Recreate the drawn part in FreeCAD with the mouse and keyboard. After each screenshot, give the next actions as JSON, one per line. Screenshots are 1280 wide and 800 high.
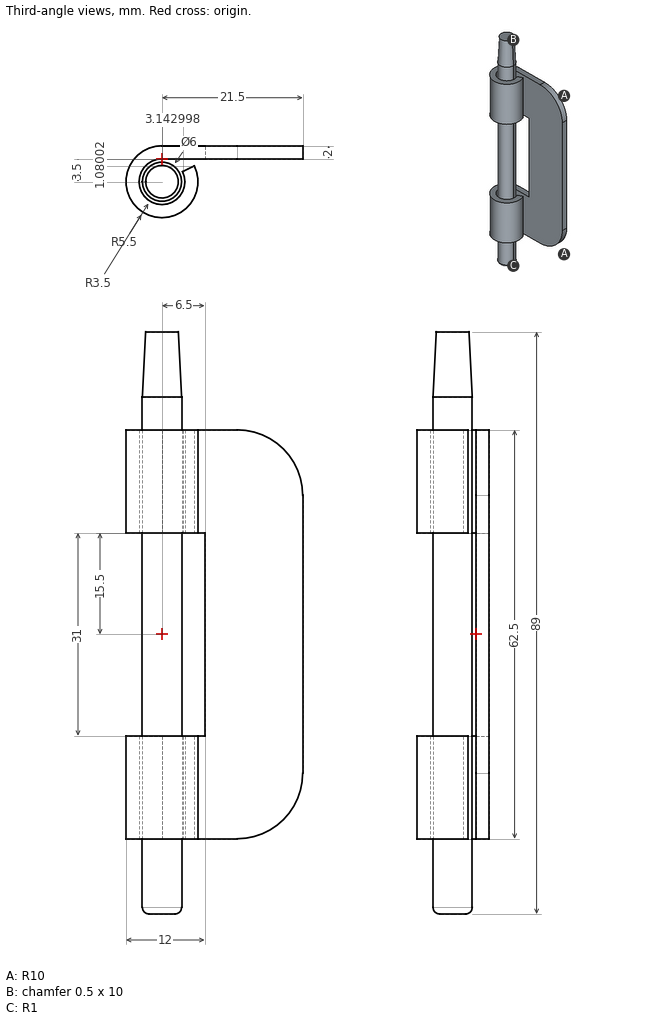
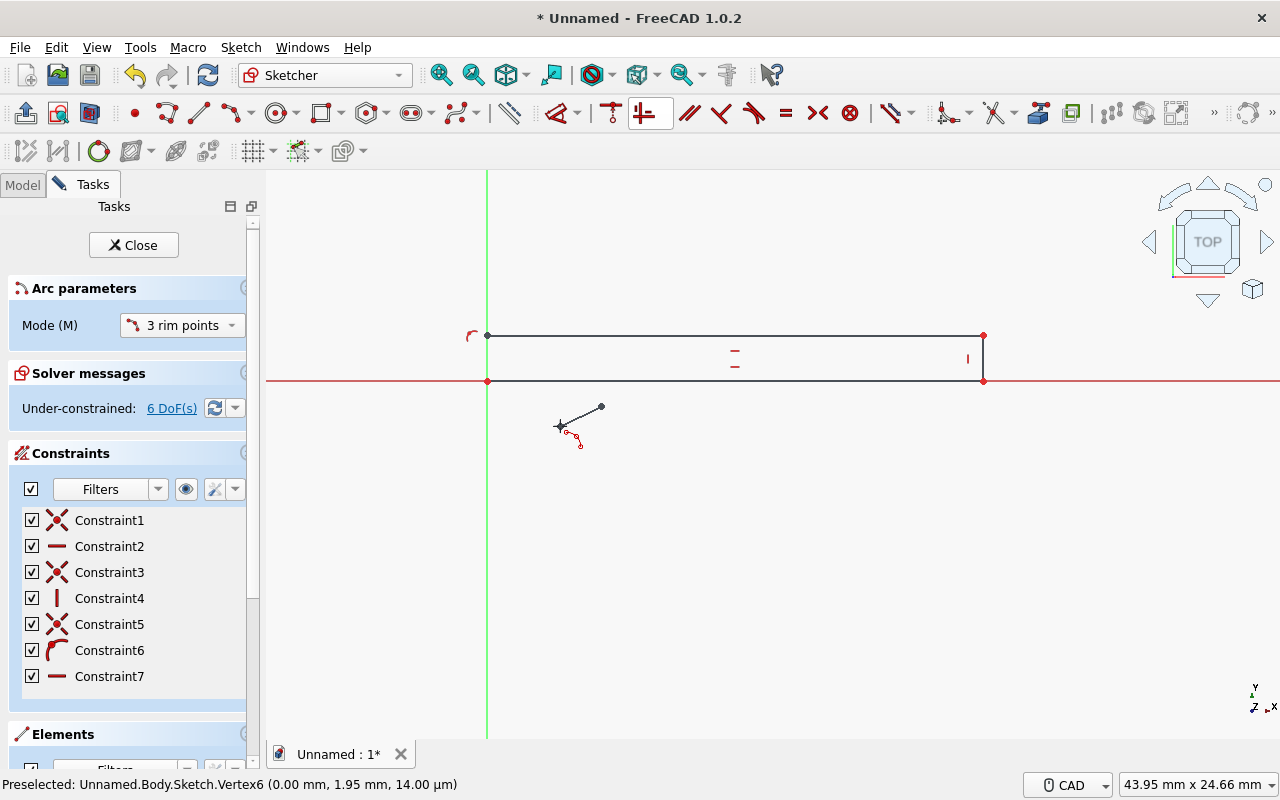
{"action": "left_click", "coordinate": [487, 336]}
{"action": "left_click", "coordinate": [601, 407]}
{"action": "left_click", "coordinate": [420, 569]}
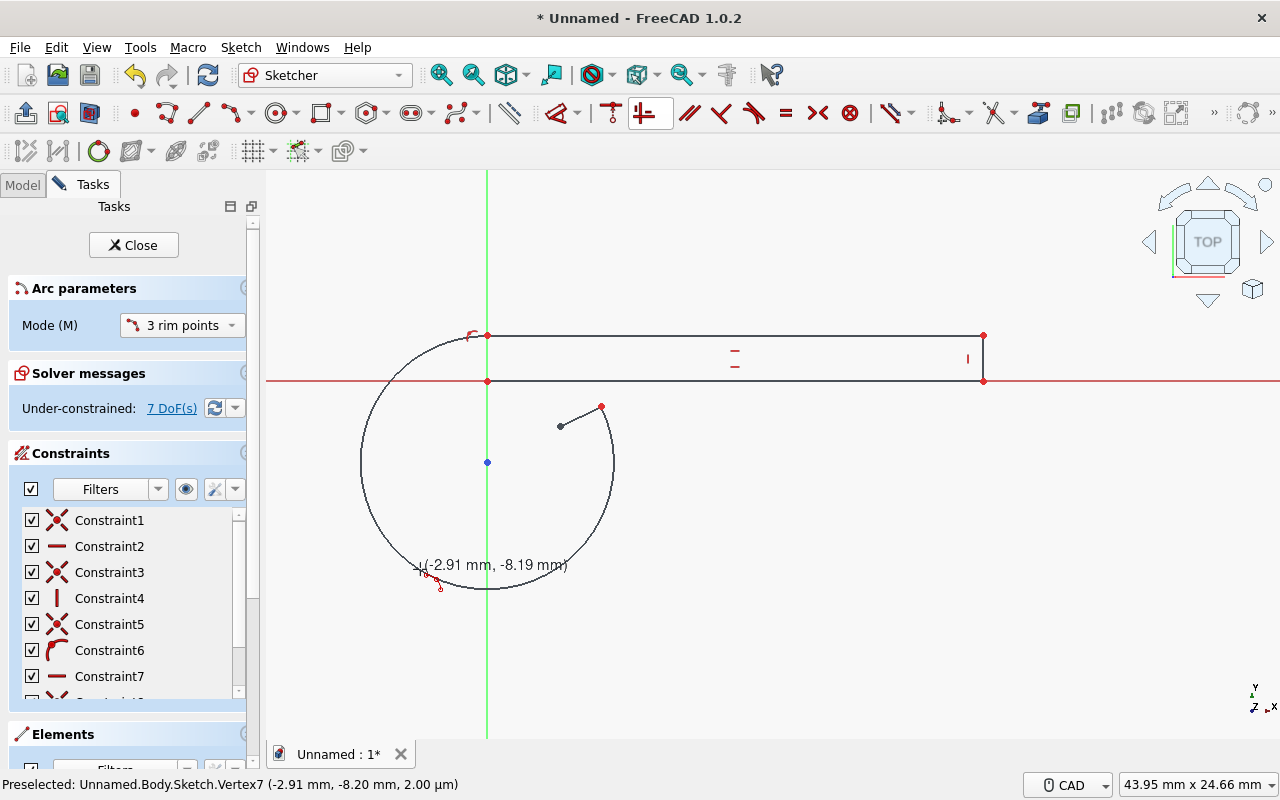
{"action": "left_click", "coordinate": [560, 427]}
{"action": "left_click", "coordinate": [487, 381]}
{"action": "left_click", "coordinate": [444, 530]}
{"action": "key", "text": "Escape"}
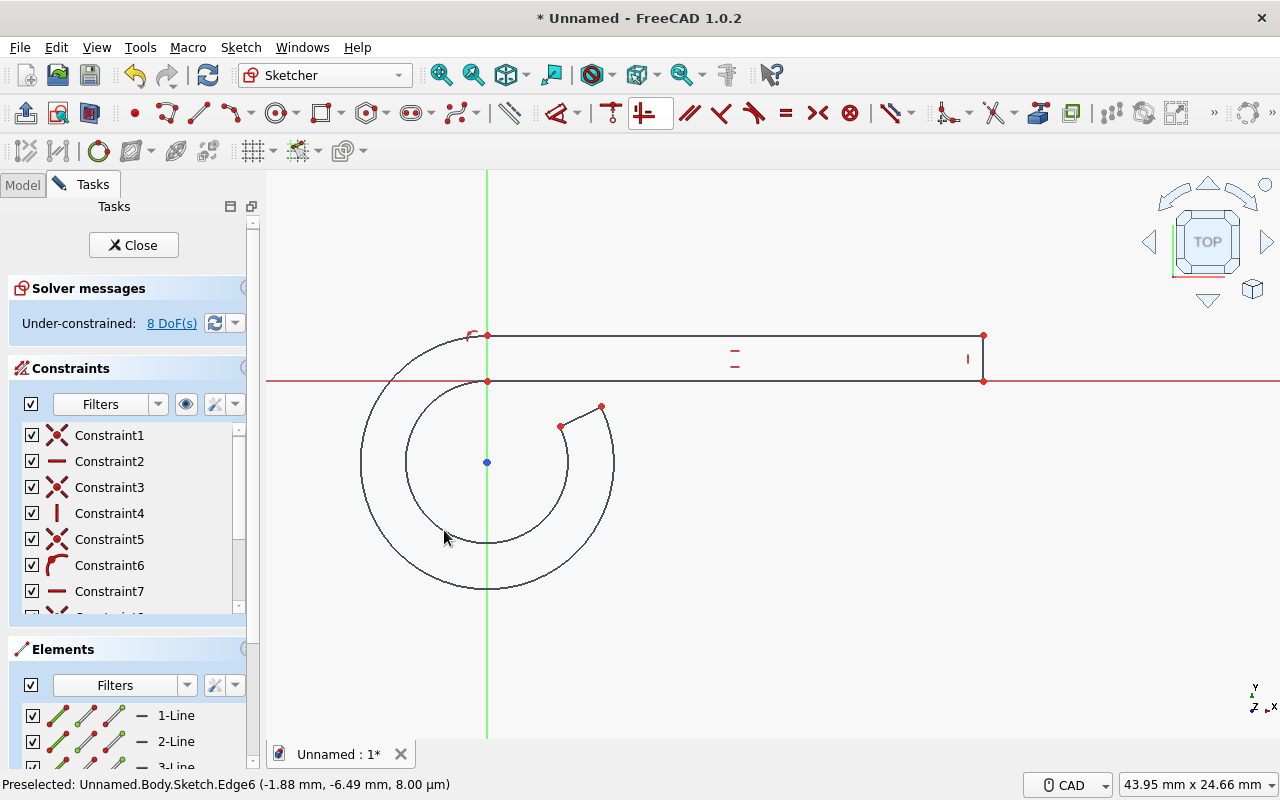
{"action": "left_click", "coordinate": [636, 381]}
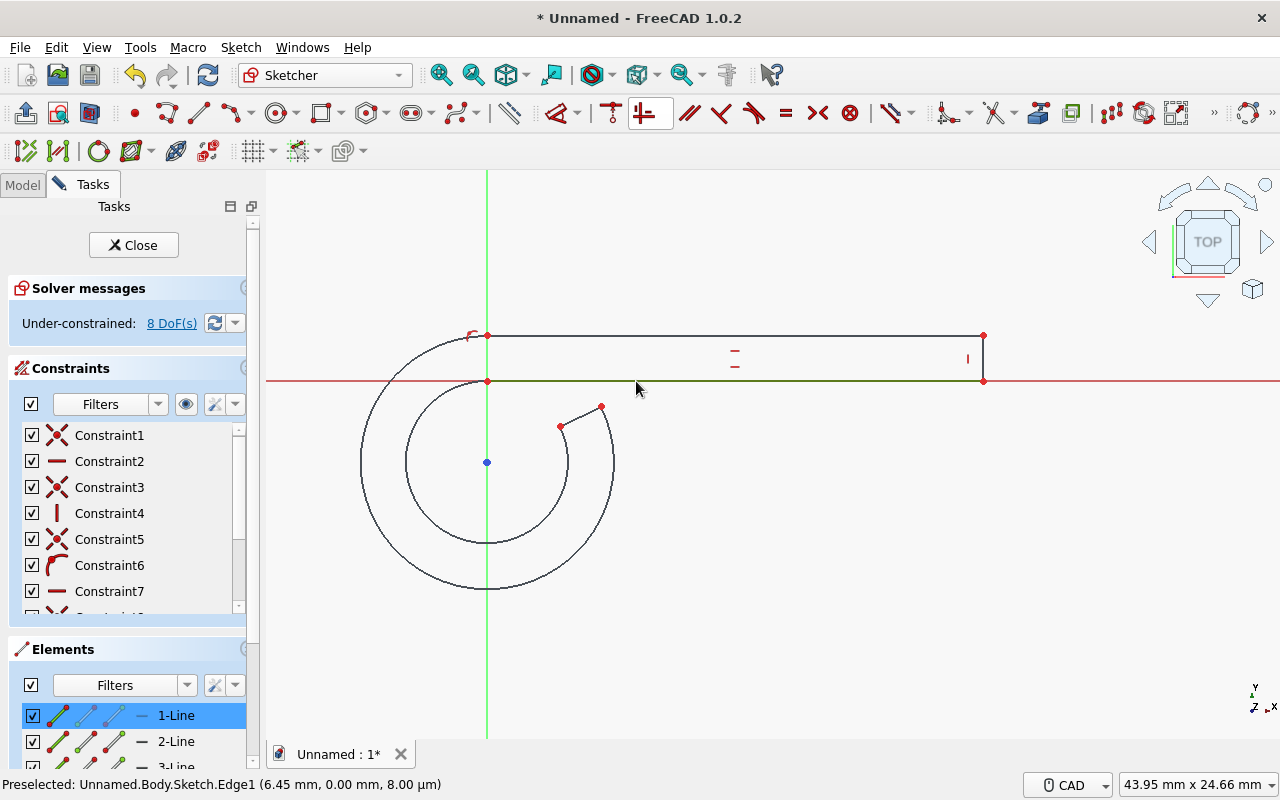
{"action": "left_click", "coordinate": [406, 460]}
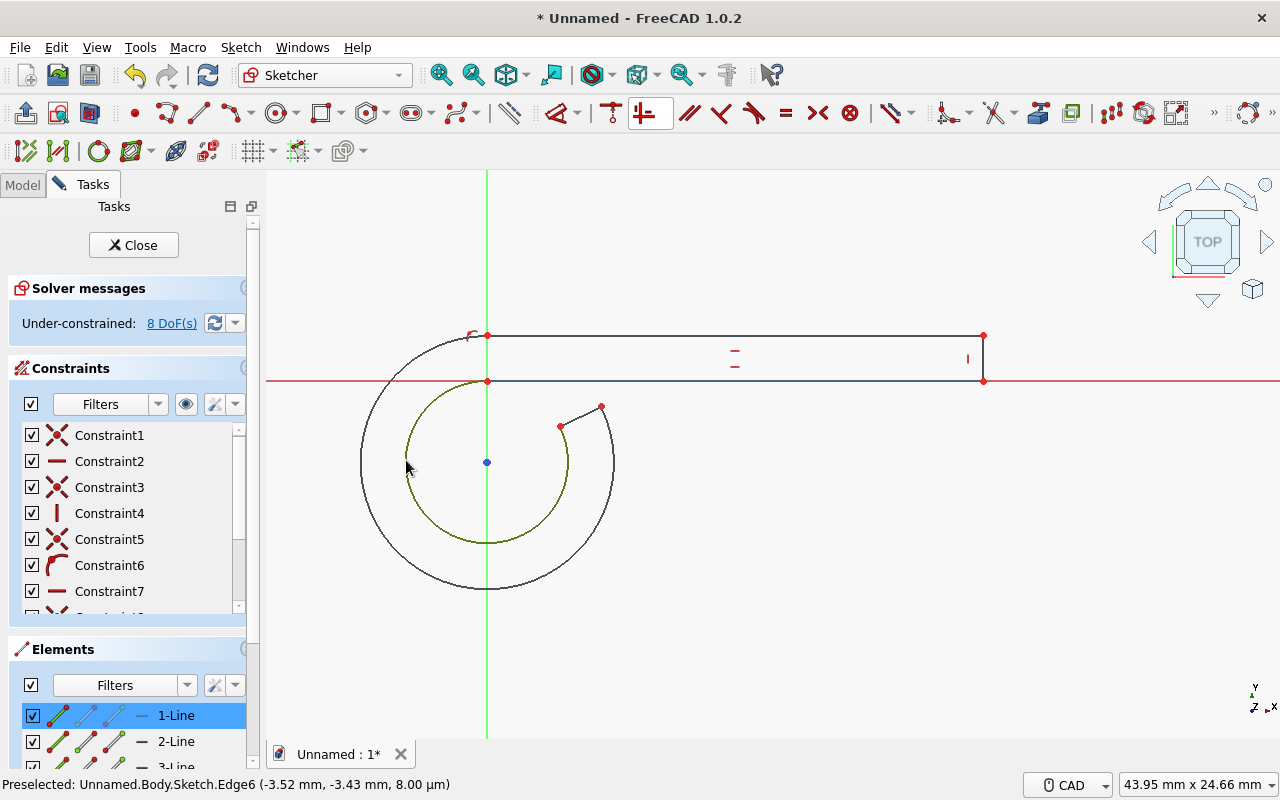
{"action": "key", "text": "t"}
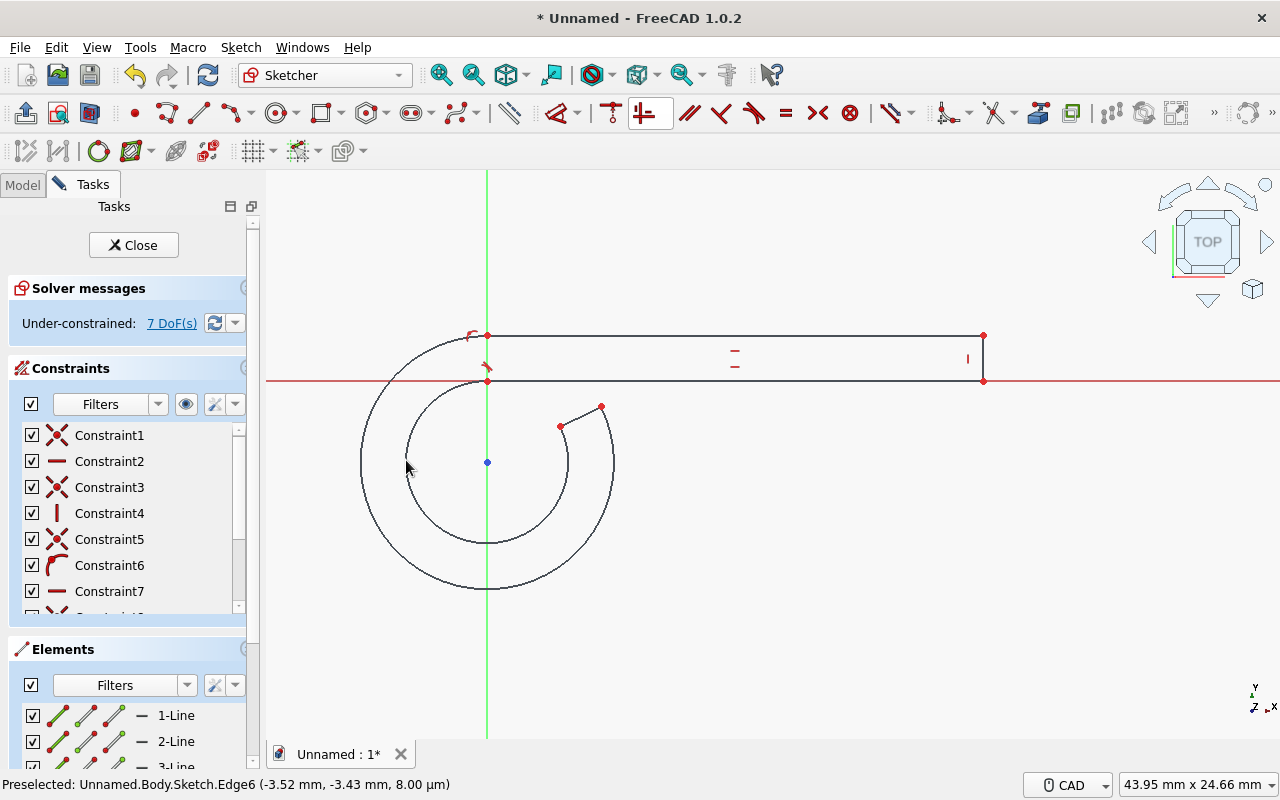
{"action": "left_click", "coordinate": [834, 336]}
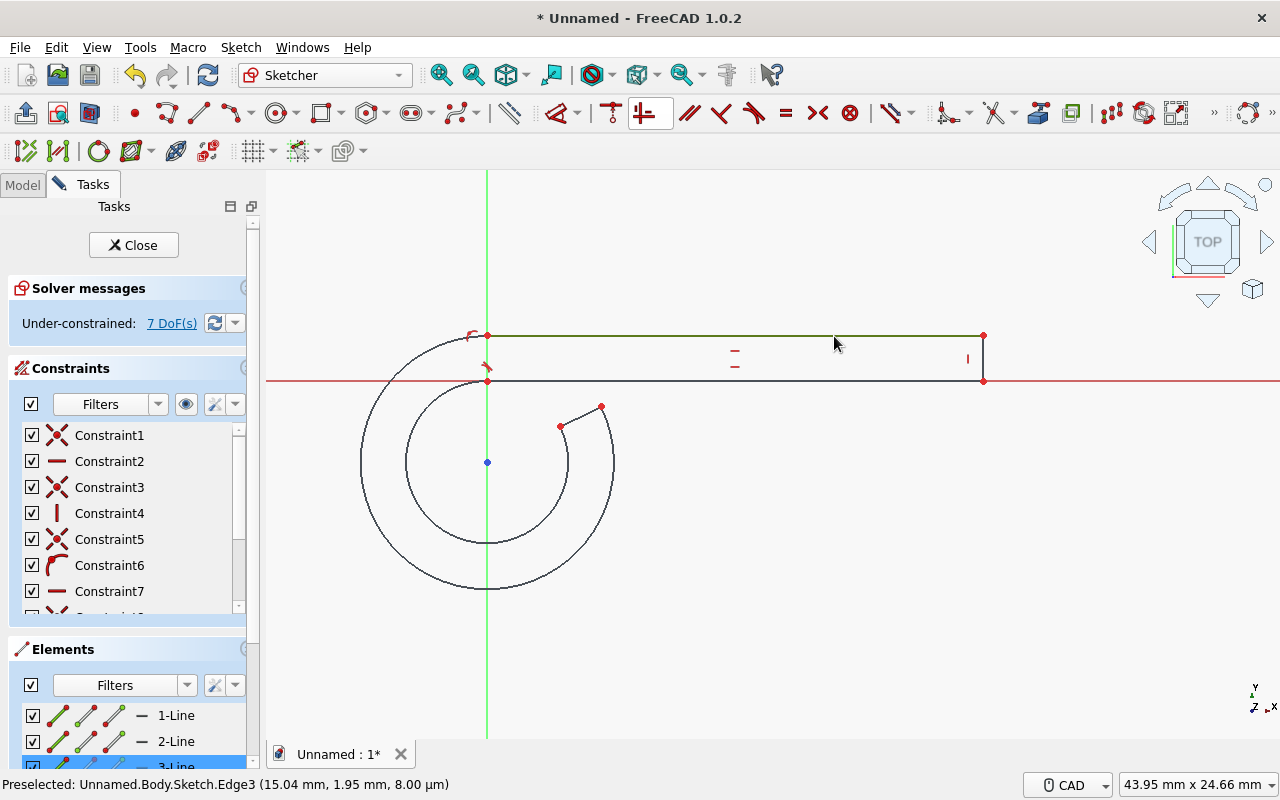
{"action": "left_click", "coordinate": [361, 460]}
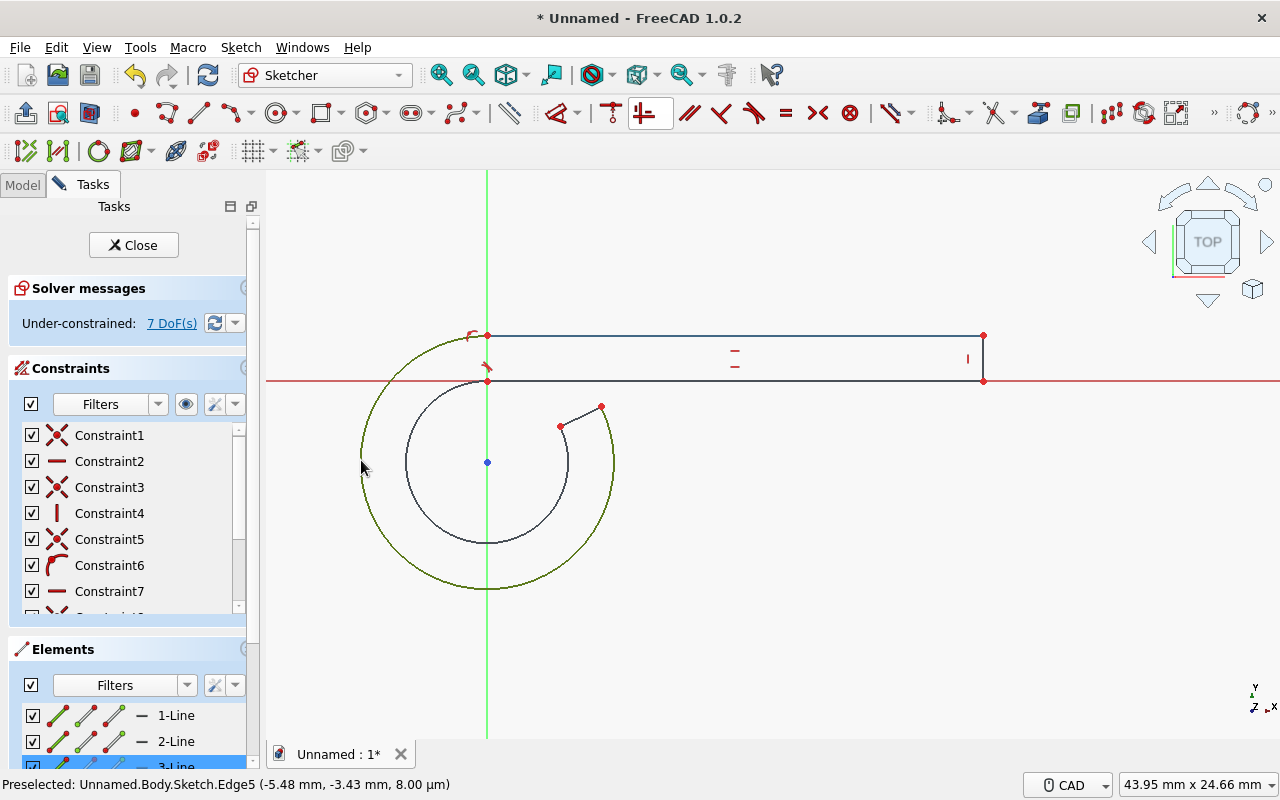
{"action": "left_click", "coordinate": [754, 114]}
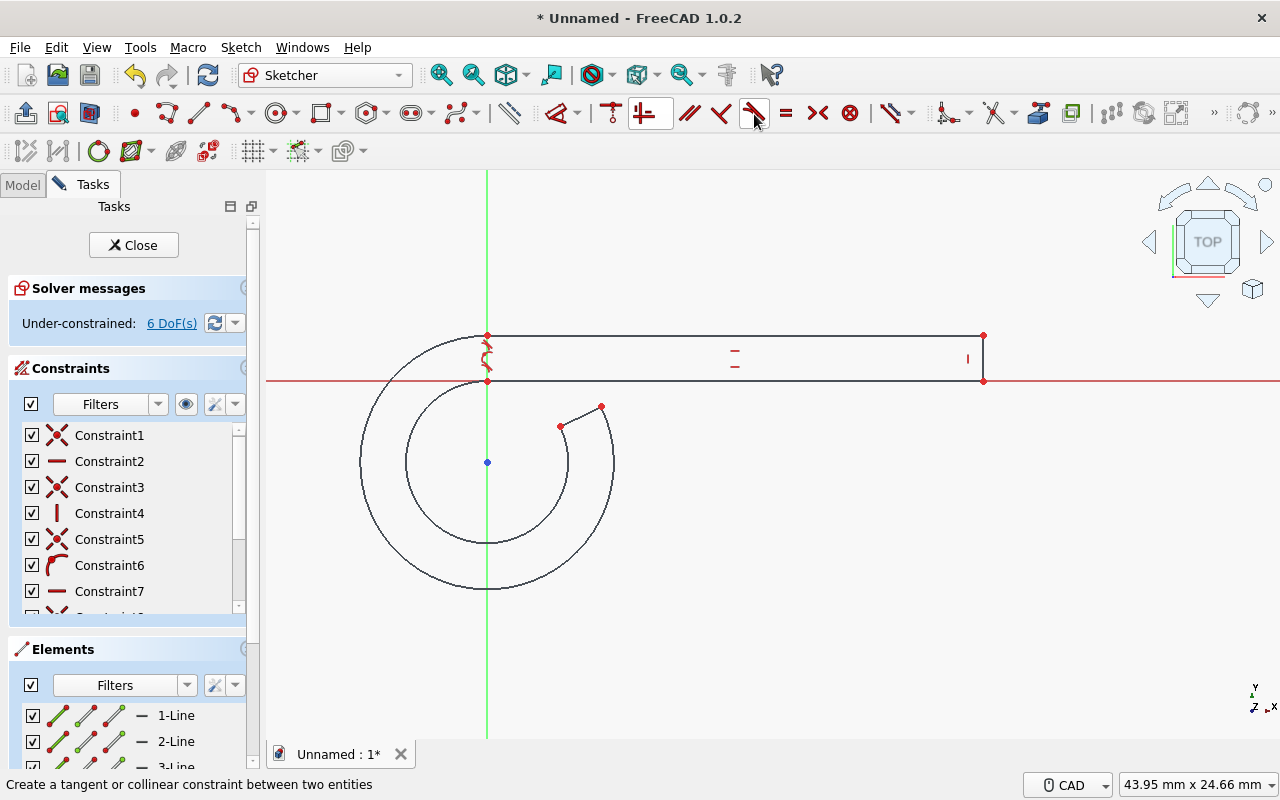
{"action": "key", "text": "d"}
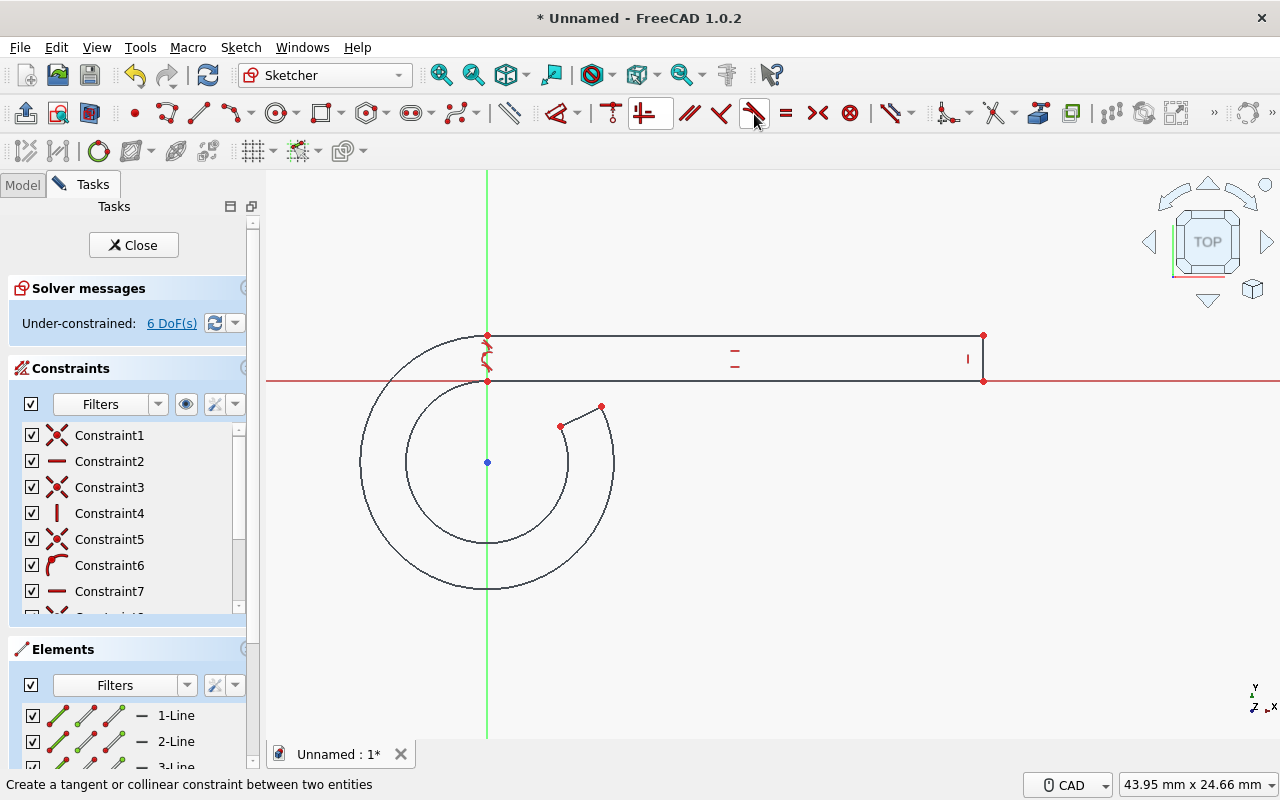
{"action": "left_click", "coordinate": [360, 460]}
{"action": "left_click", "coordinate": [328, 459]}